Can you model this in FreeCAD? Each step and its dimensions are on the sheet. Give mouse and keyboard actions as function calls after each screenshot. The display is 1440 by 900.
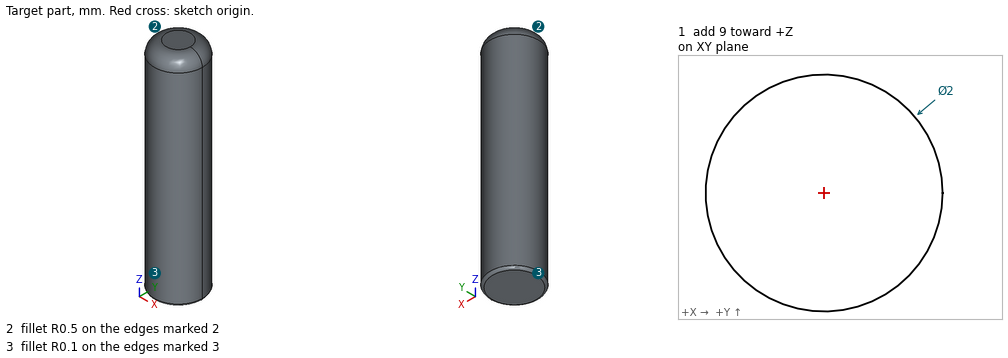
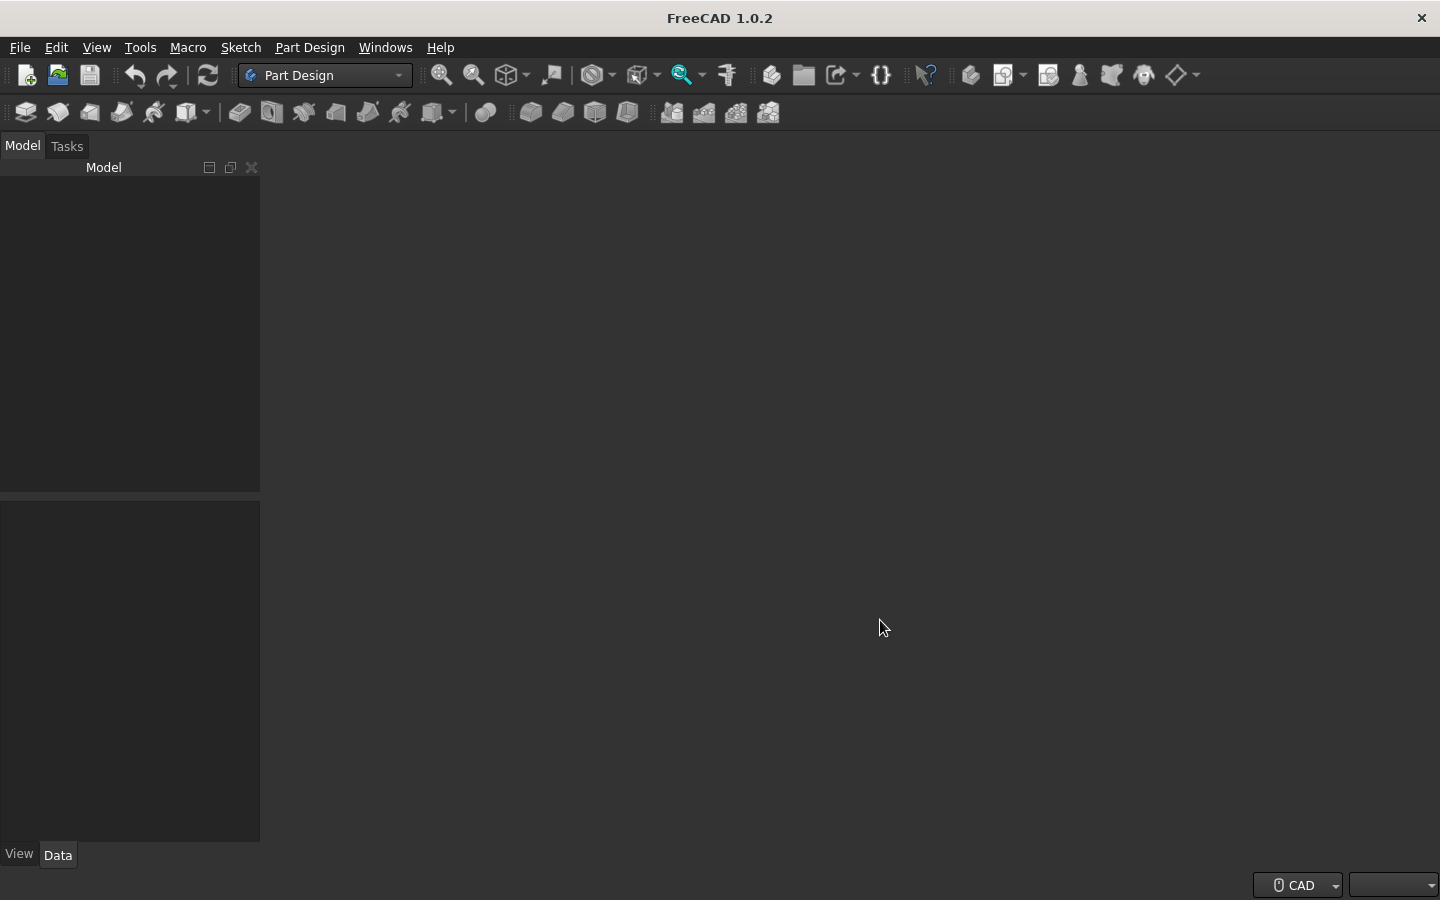
click(26, 76)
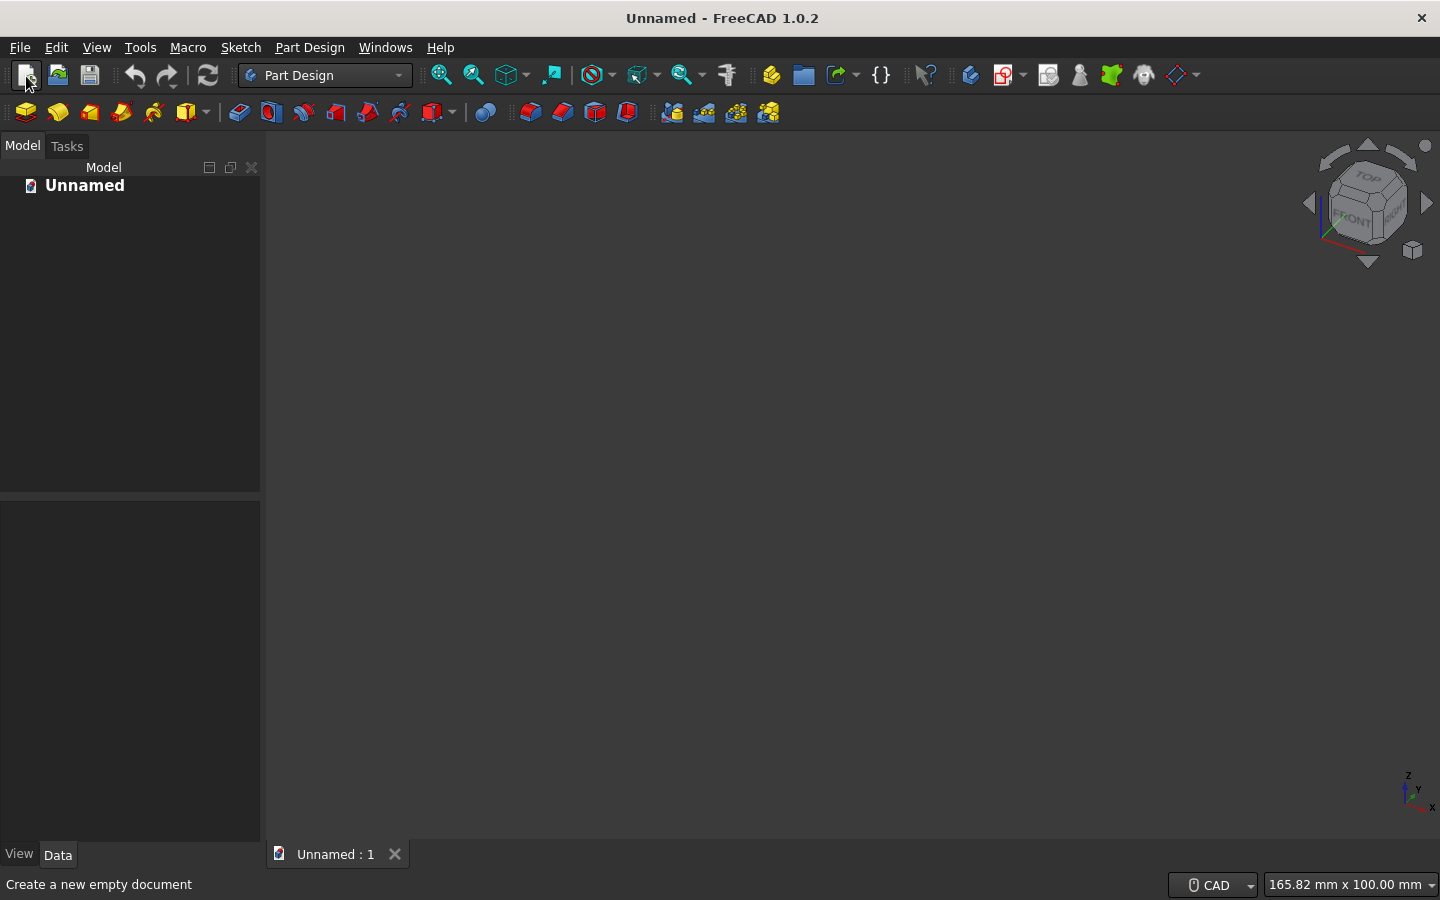
click(1004, 76)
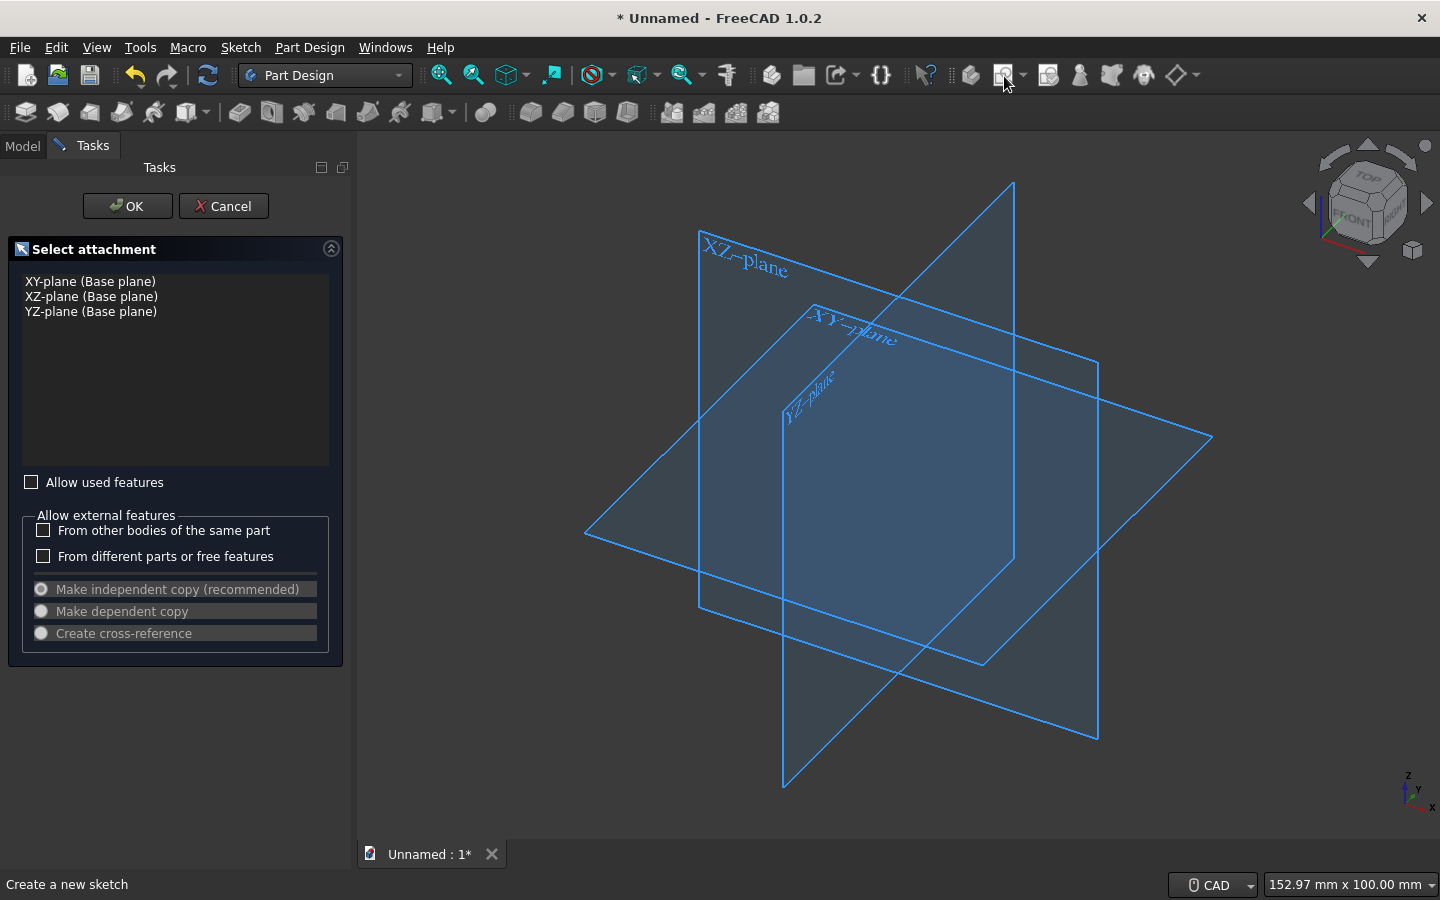
click(82, 282)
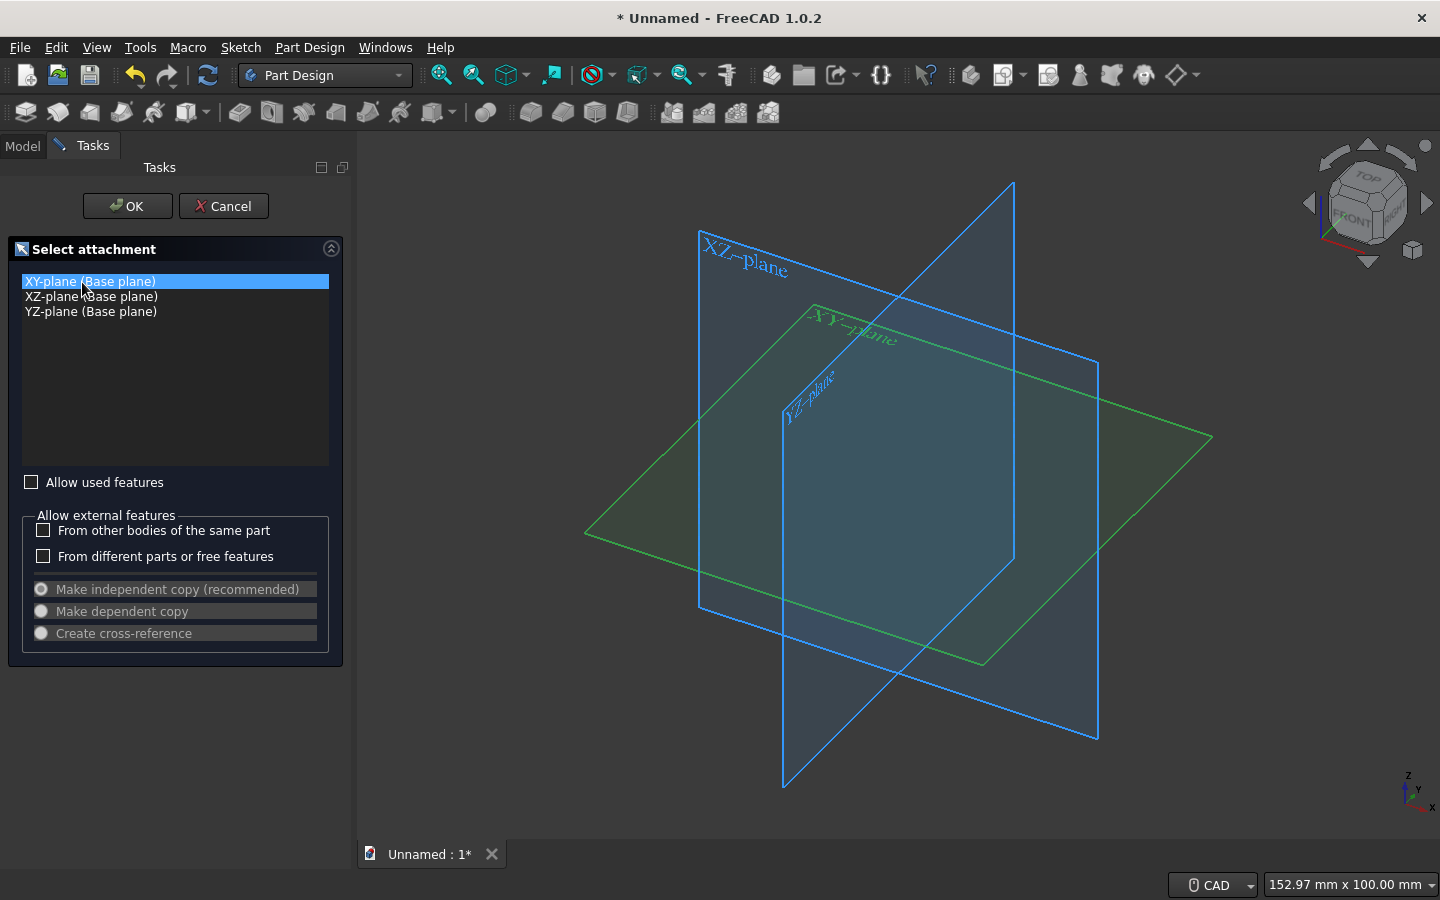
click(128, 206)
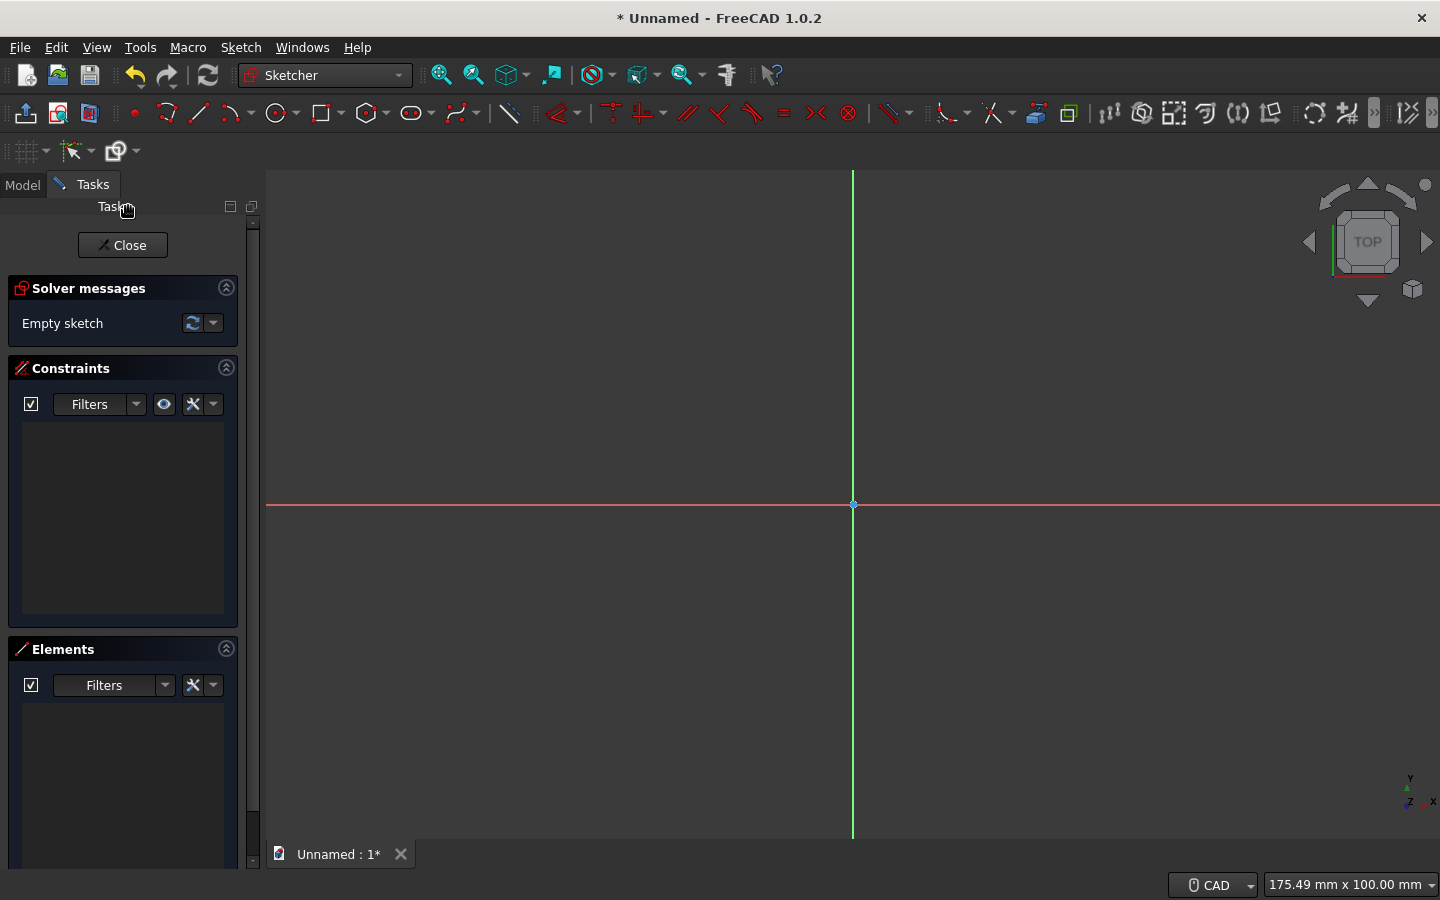
scroll(857, 504, up, 15)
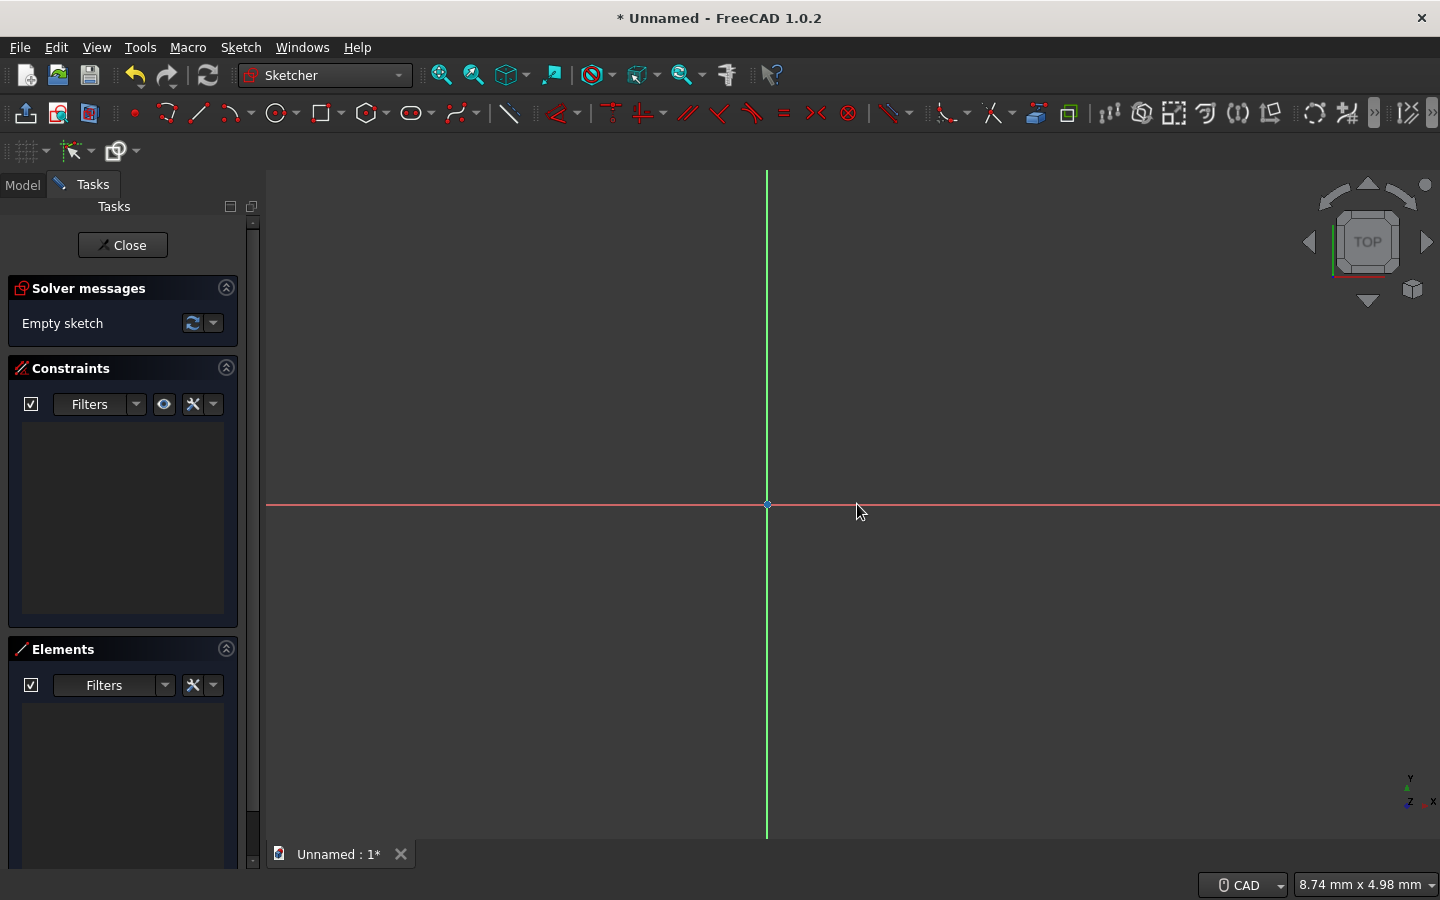
scroll(732, 504, up, 2)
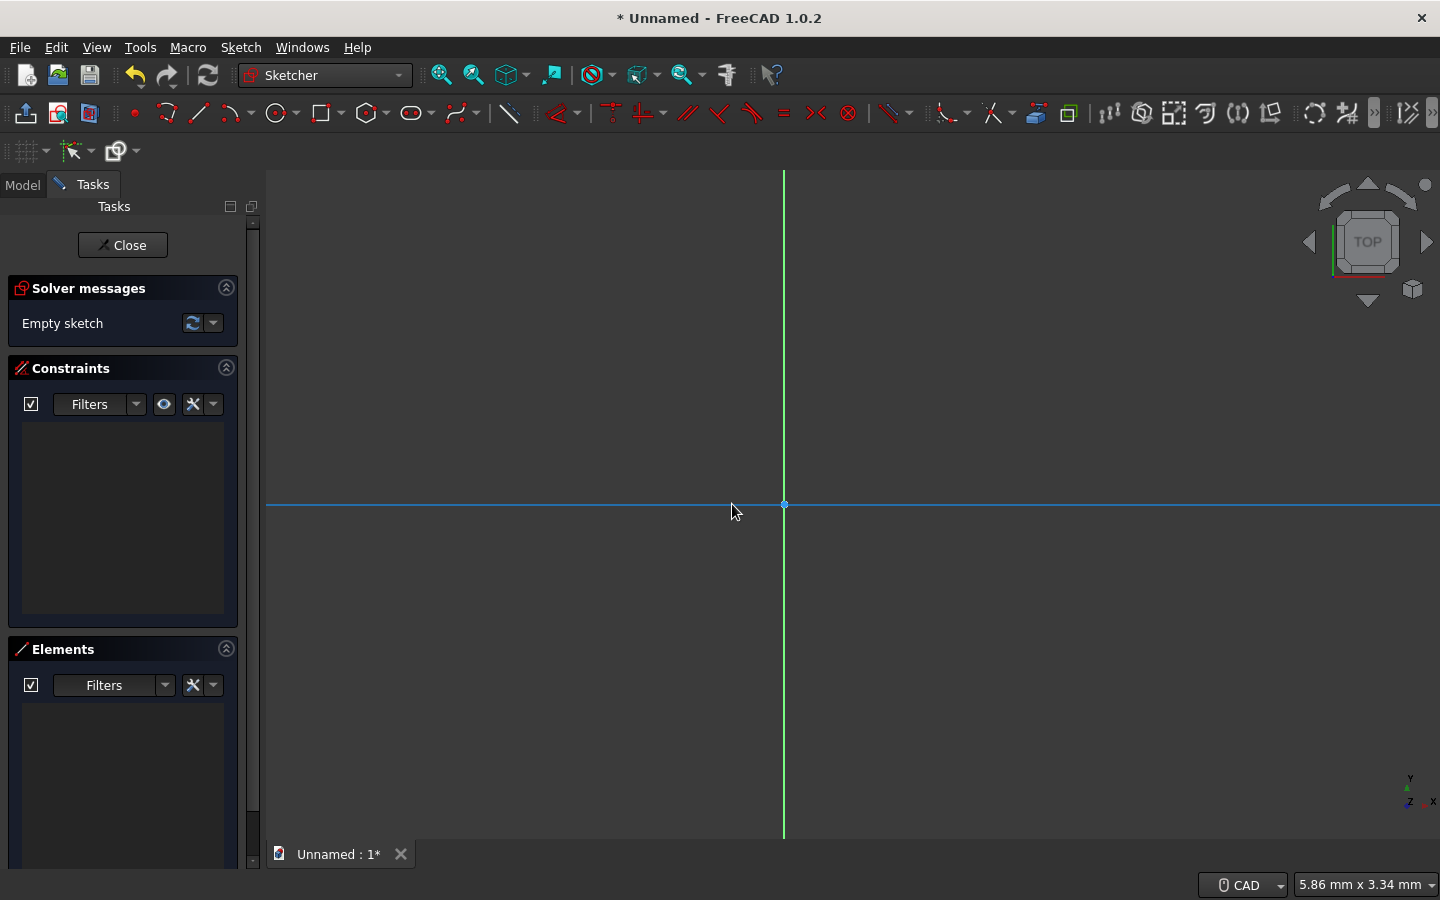
click(276, 114)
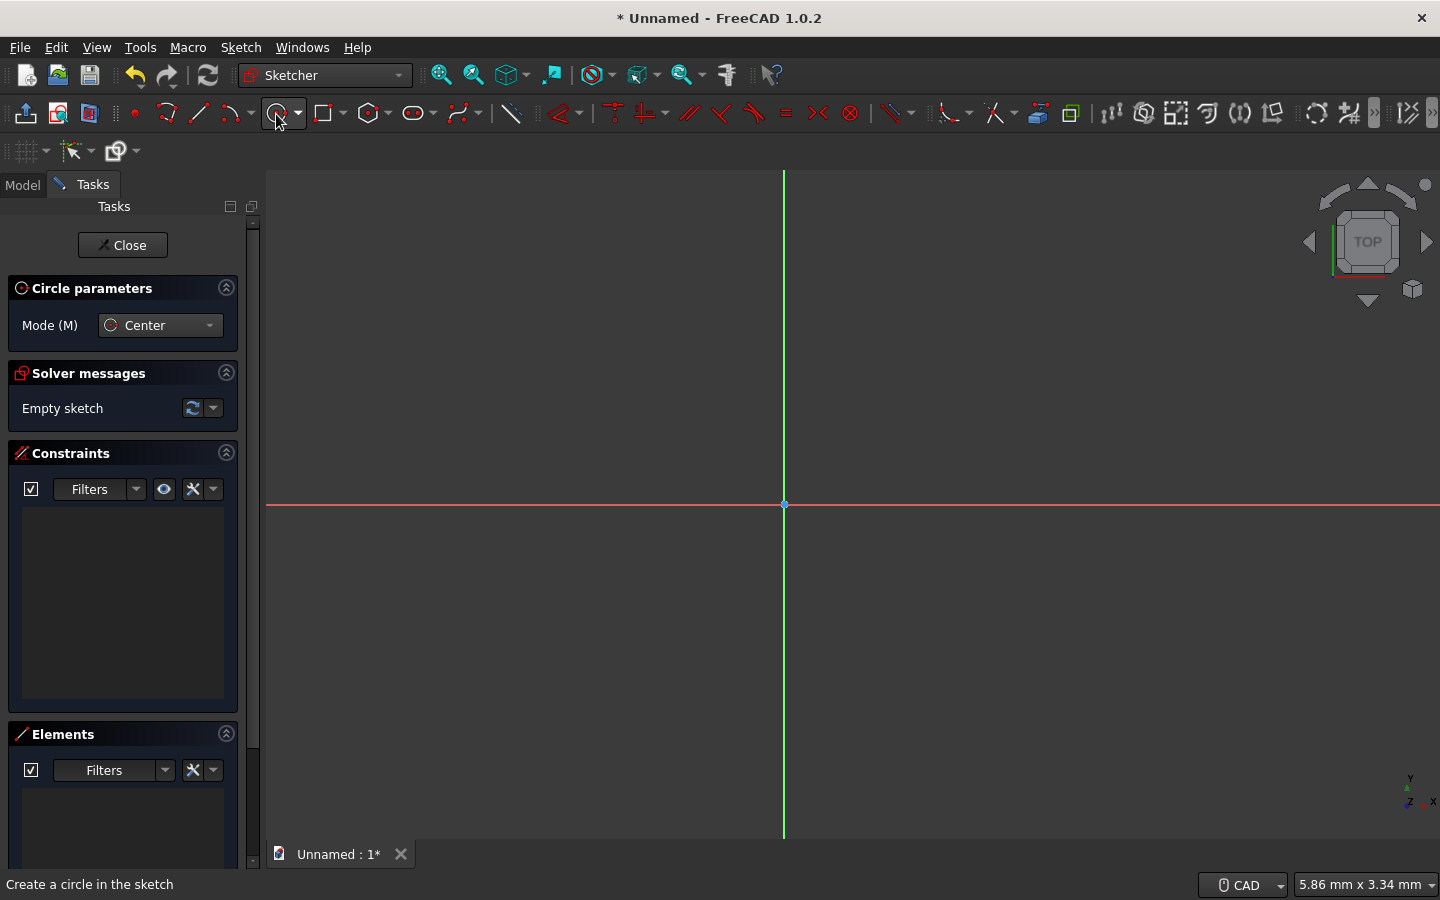
click(784, 504)
click(926, 363)
key(Escape)